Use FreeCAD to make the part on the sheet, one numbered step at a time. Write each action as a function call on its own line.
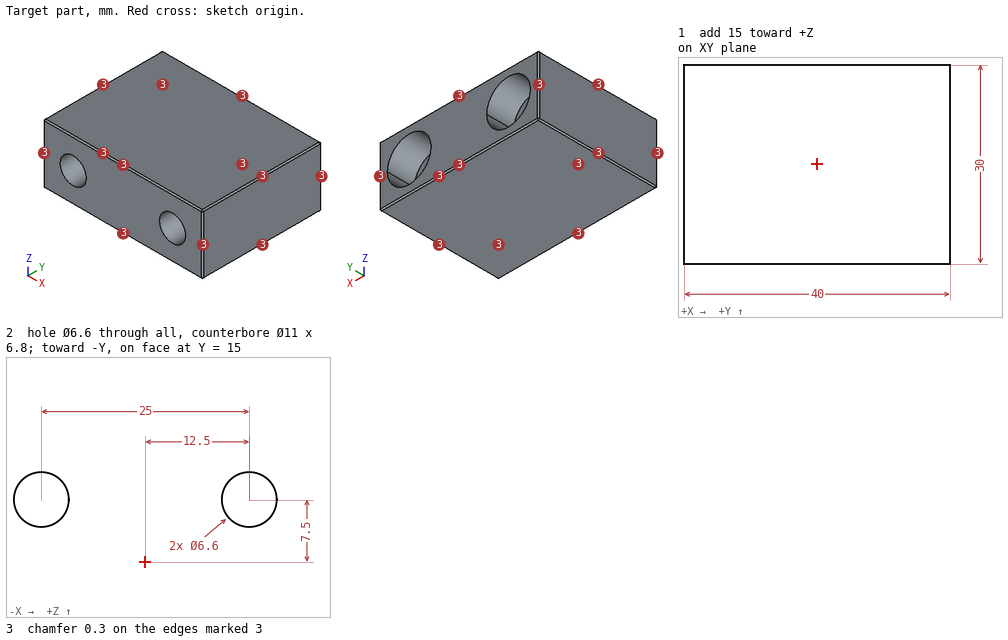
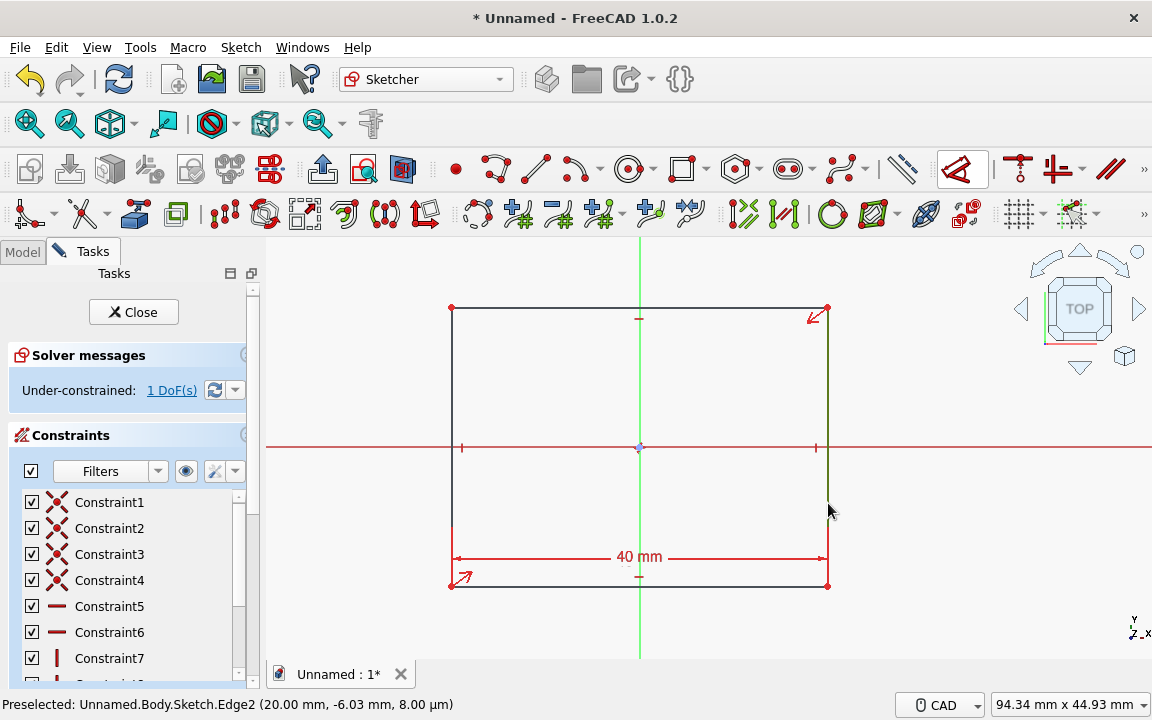
click(982, 170)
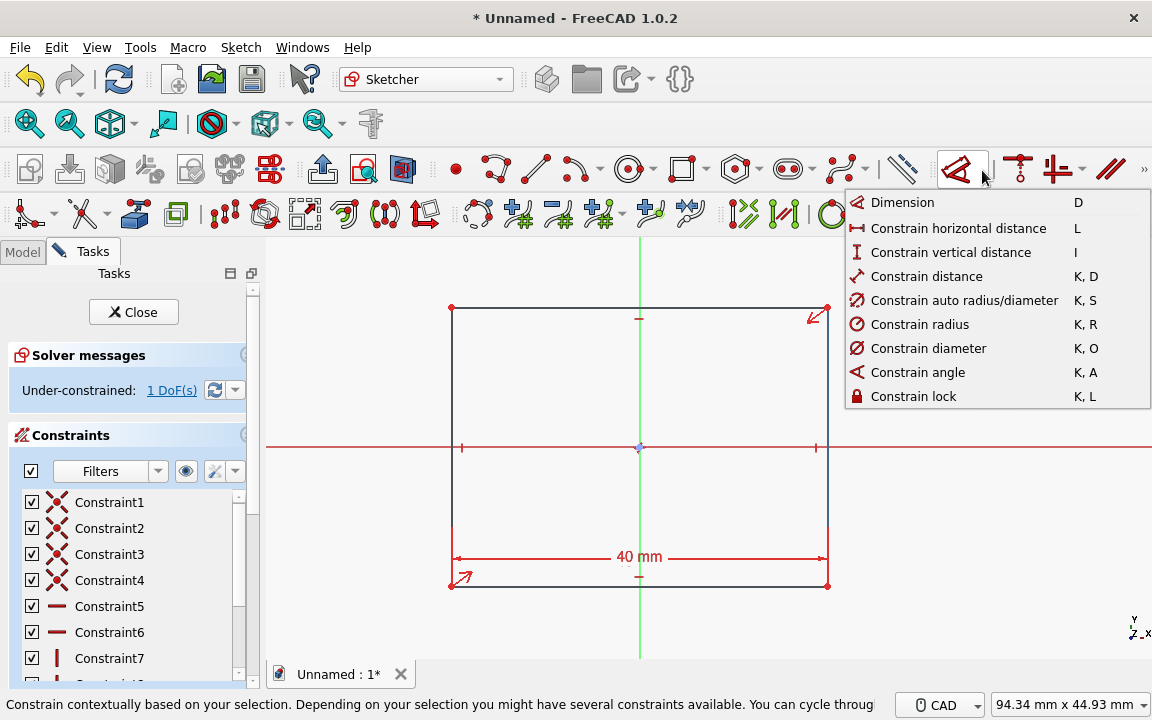
click(998, 252)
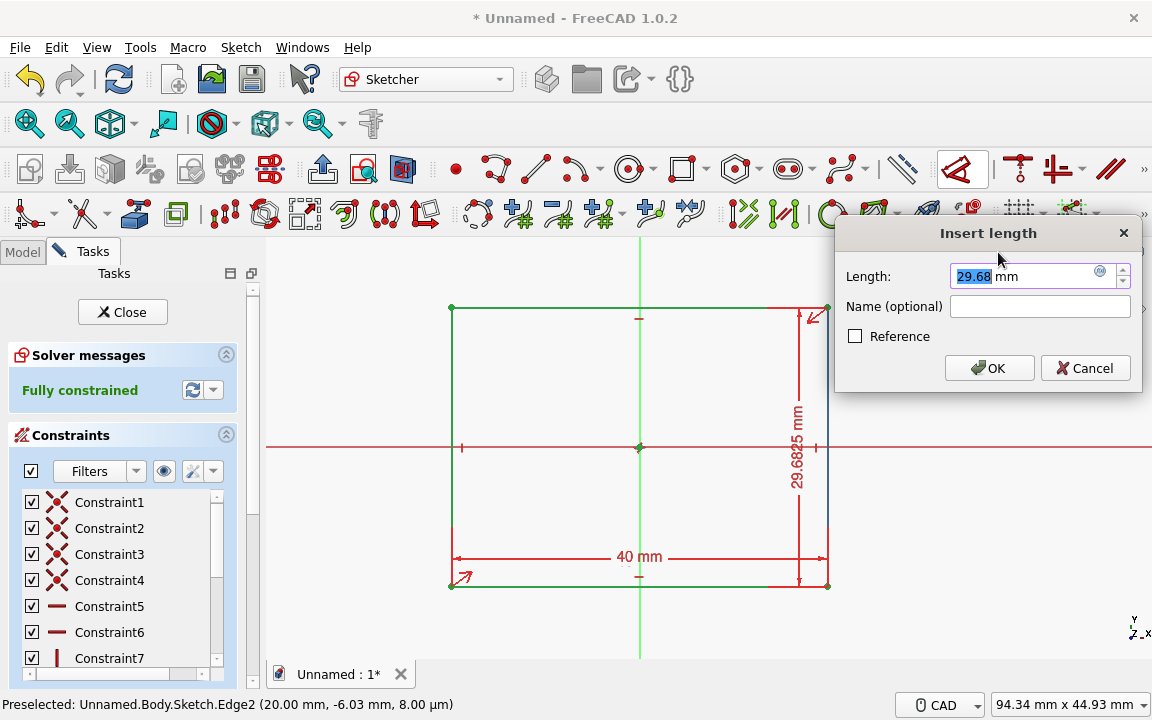
text(30)
key(Return)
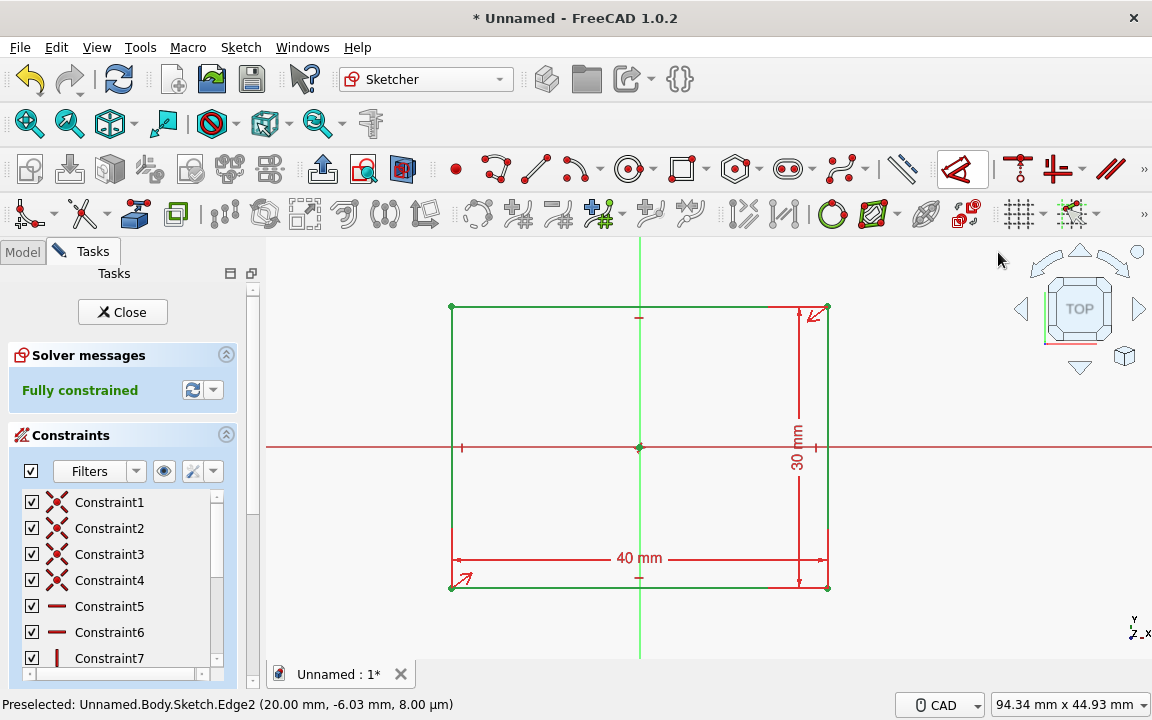
click(123, 312)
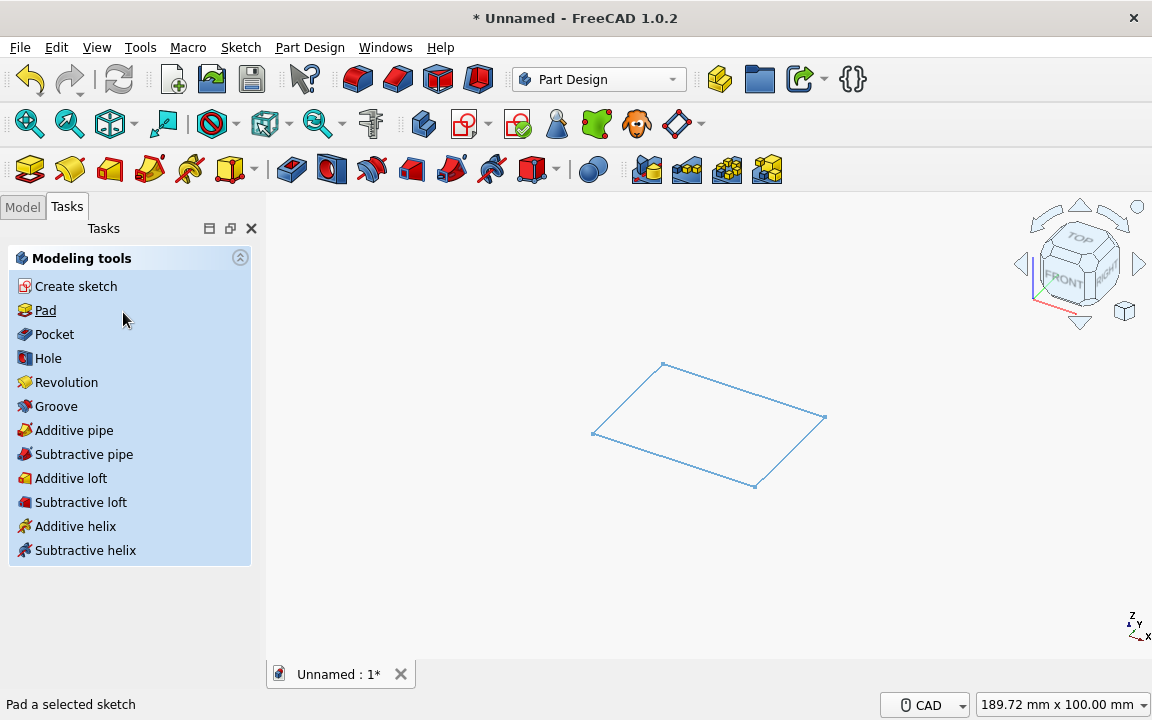
click(30, 170)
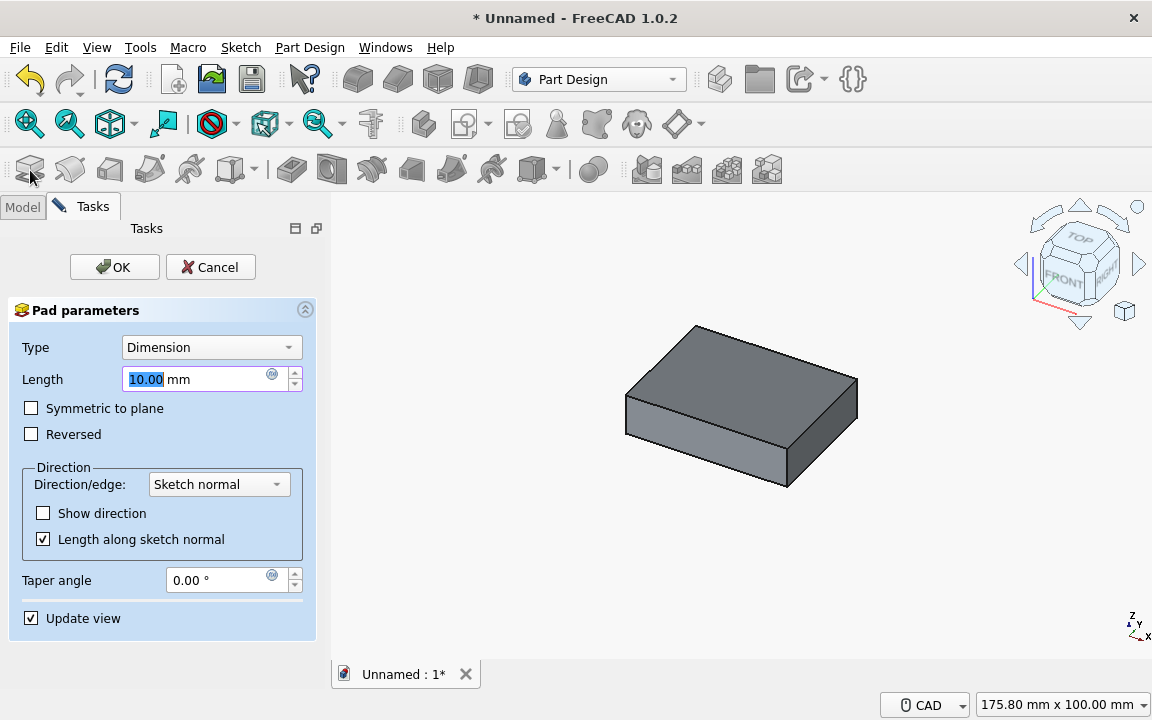
text(15)
key(Tab)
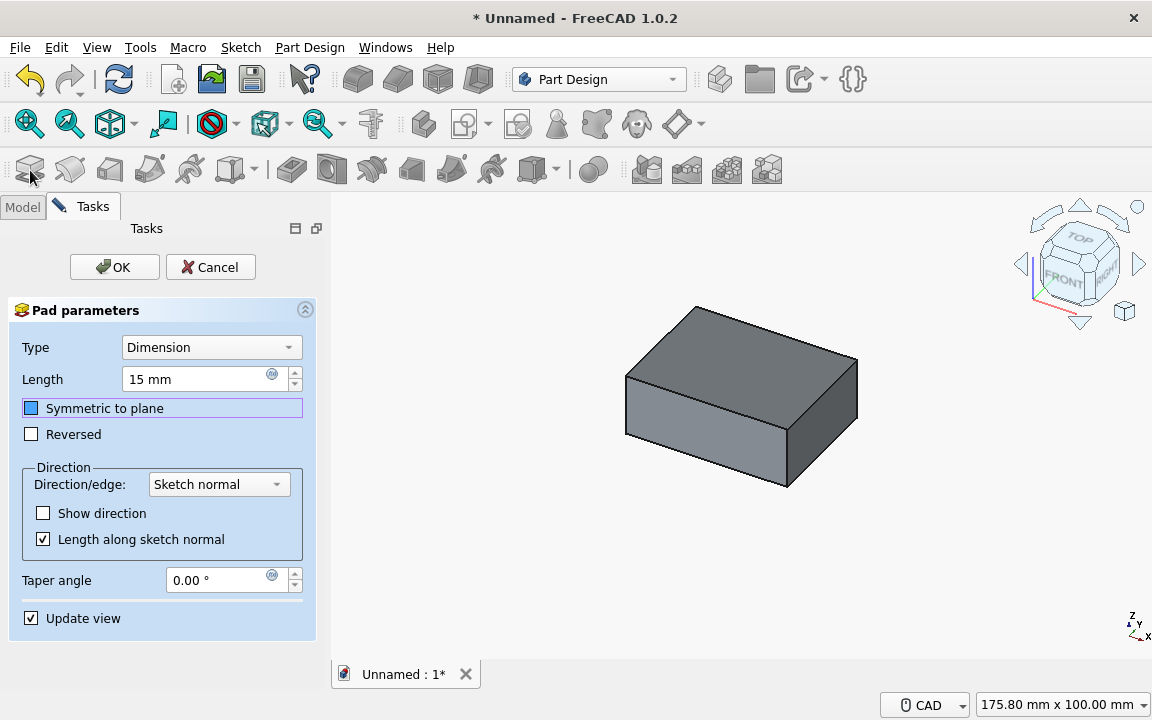
click(115, 267)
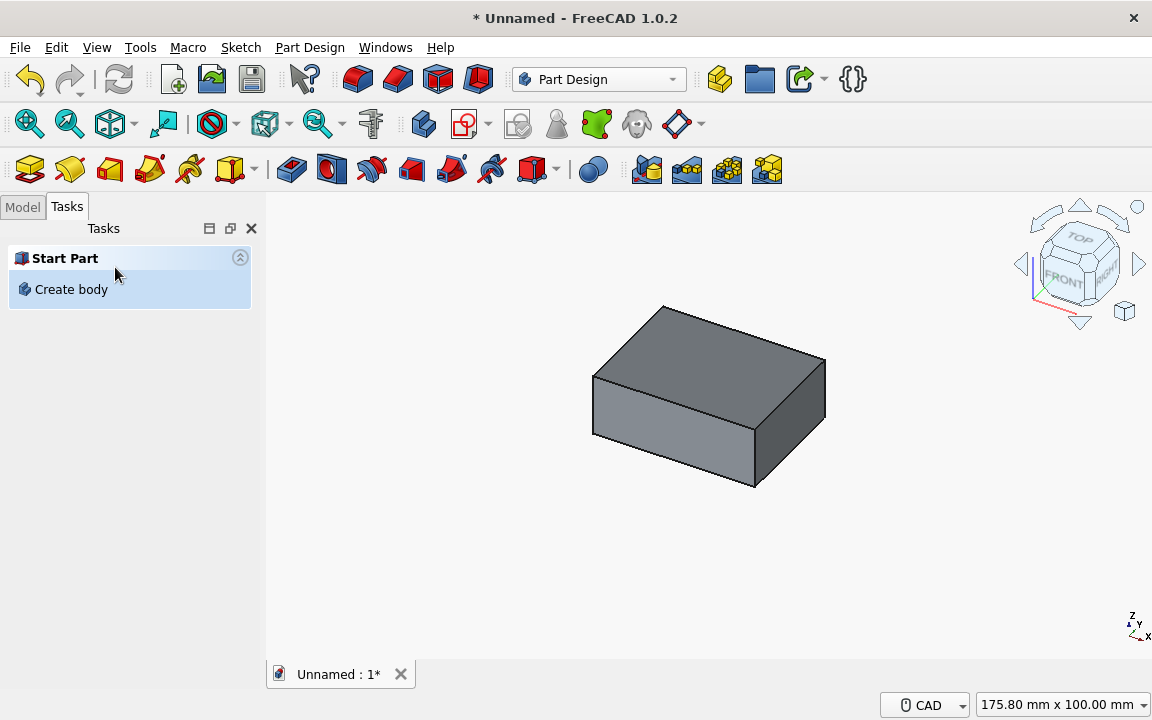
click(30, 124)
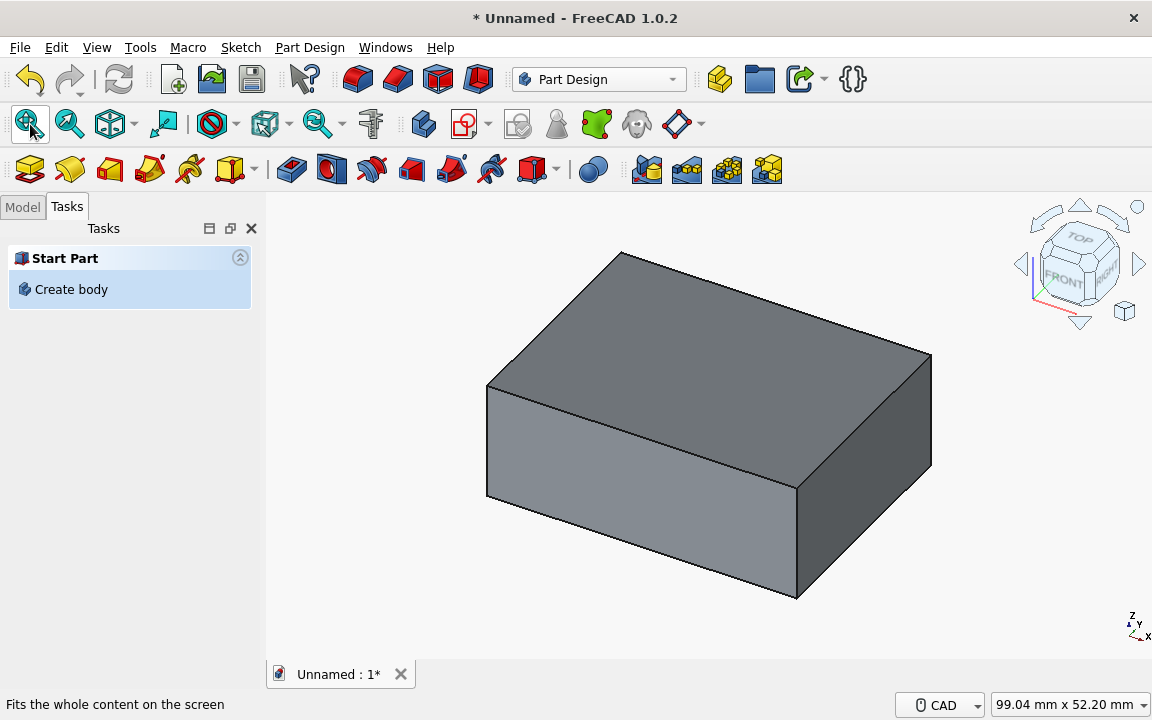
key(4)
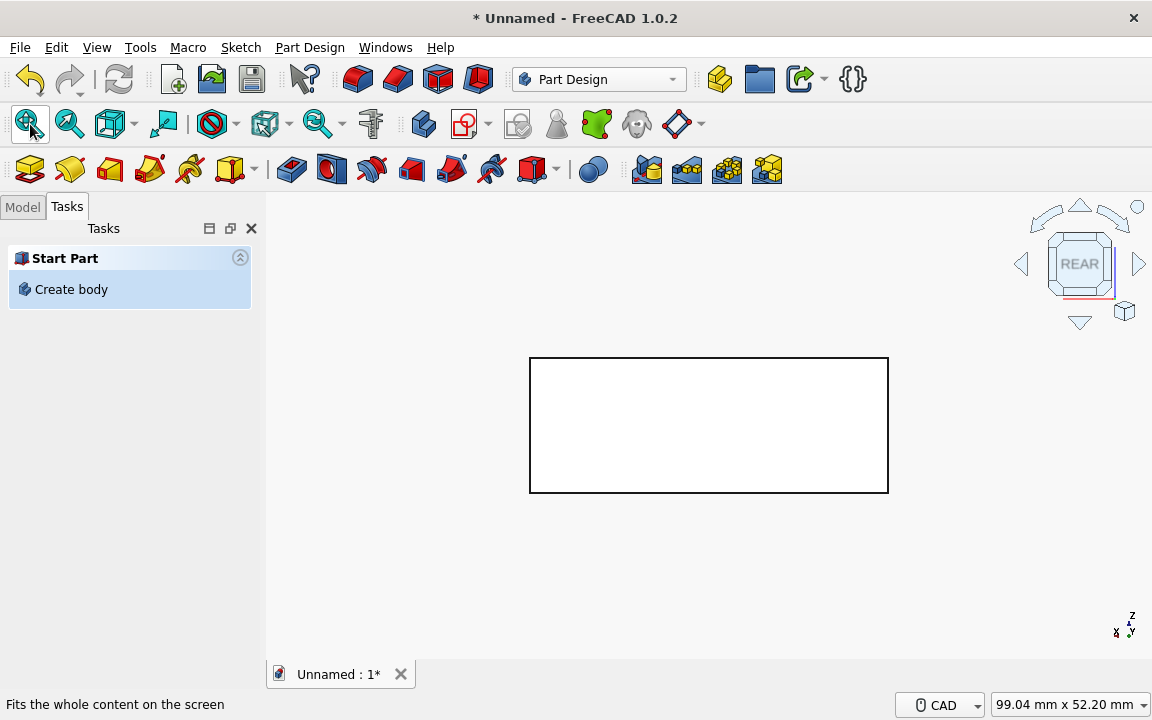
click(30, 124)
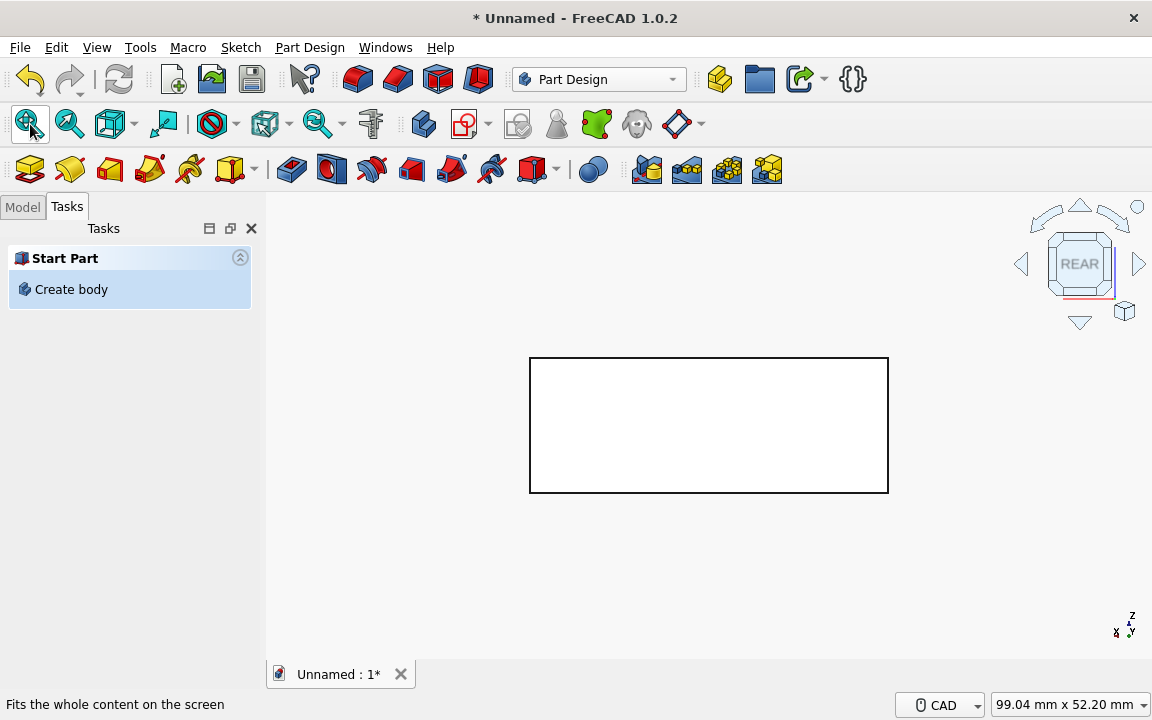
click(607, 425)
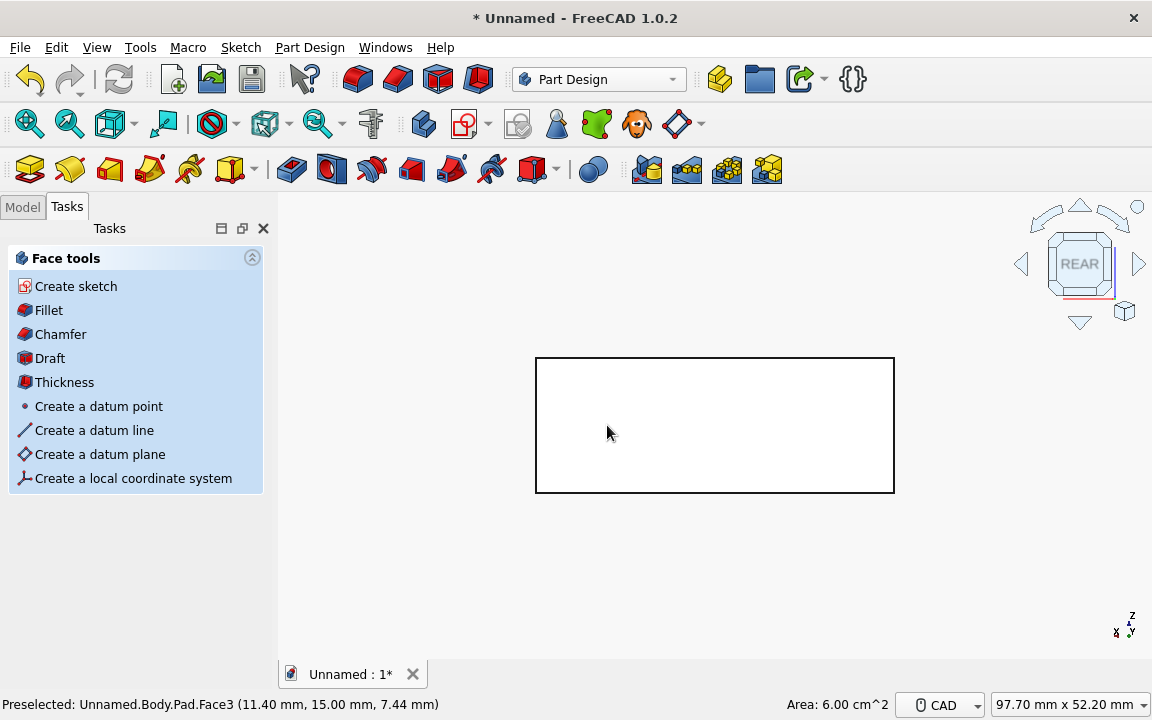
click(464, 124)